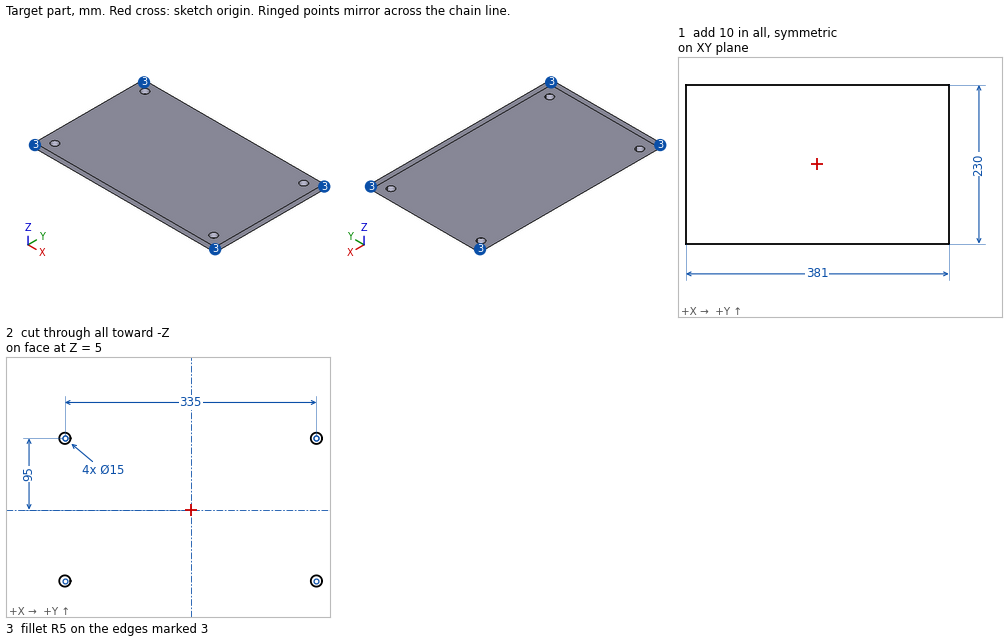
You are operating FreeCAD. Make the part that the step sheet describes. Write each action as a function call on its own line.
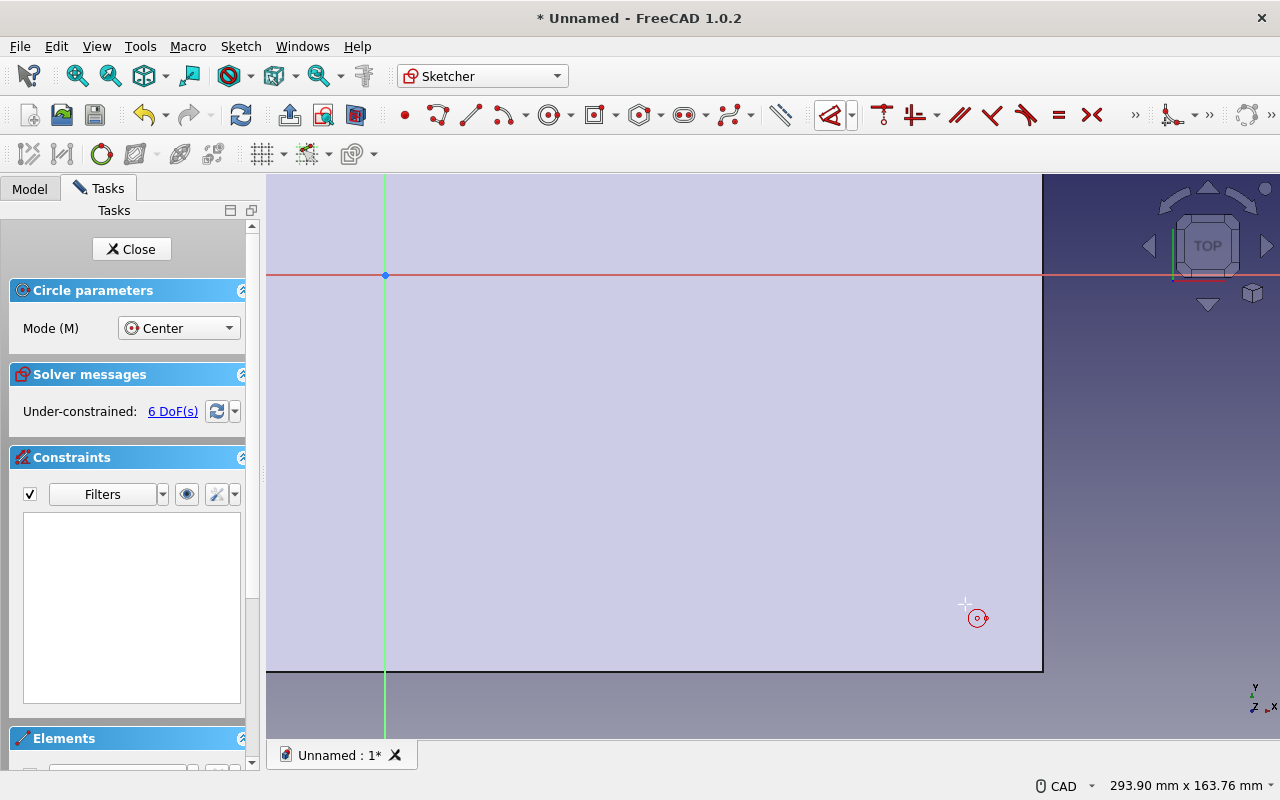
click(963, 603)
click(981, 585)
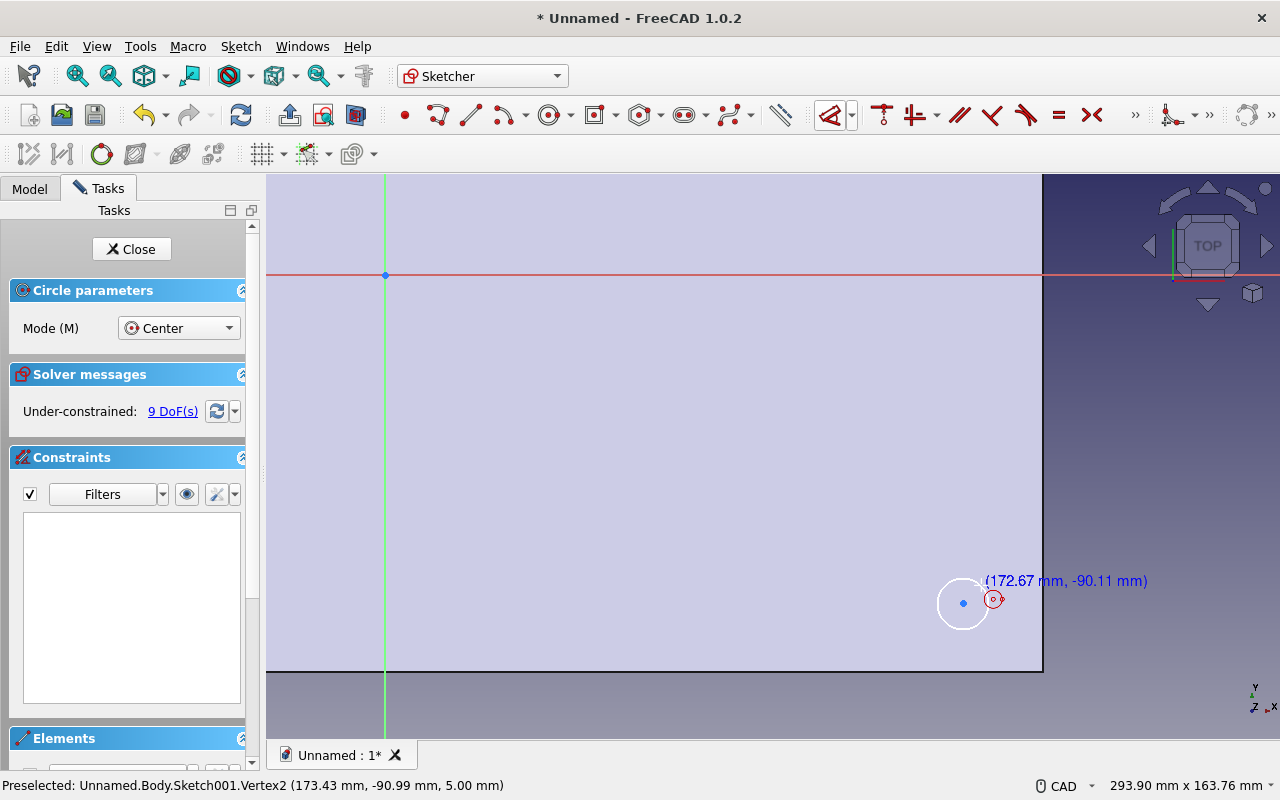
scroll(965, 605, down, 4)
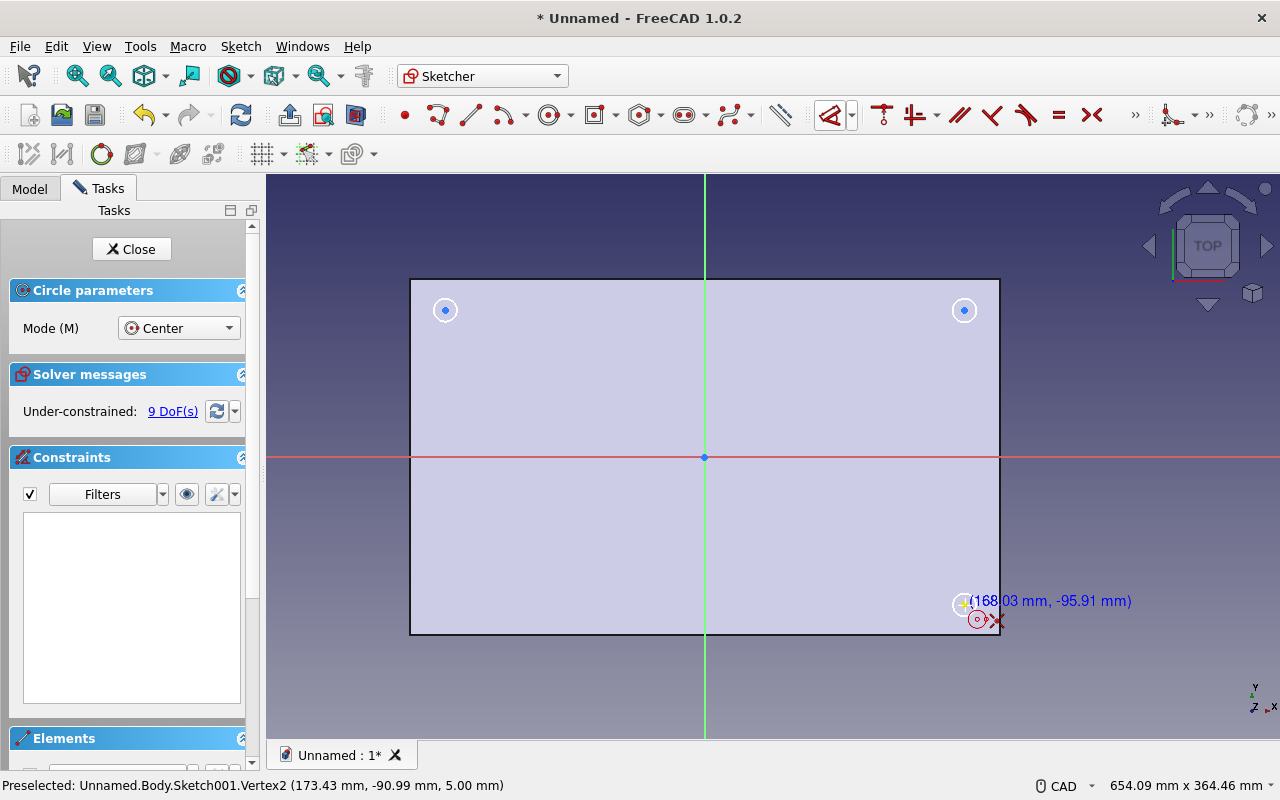
scroll(445, 604, up, 4)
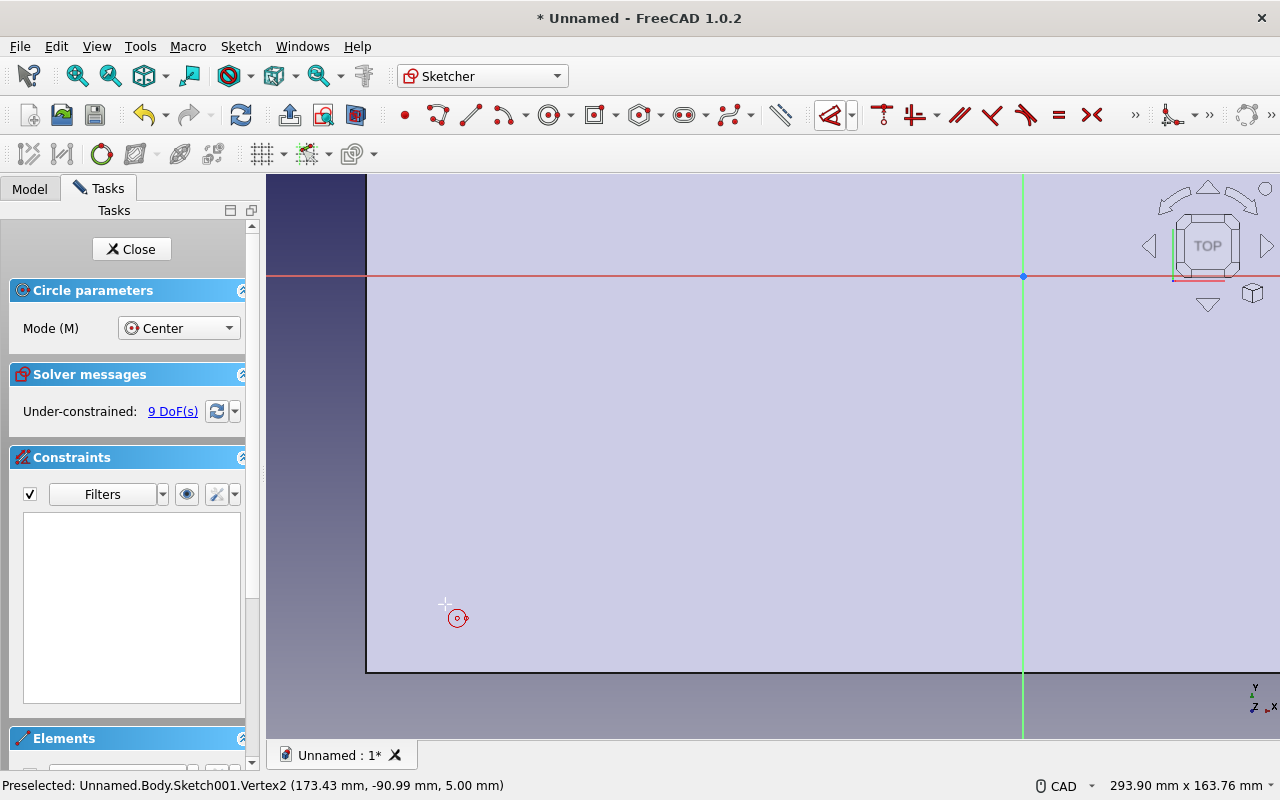
click(445, 604)
click(464, 586)
key(Escape)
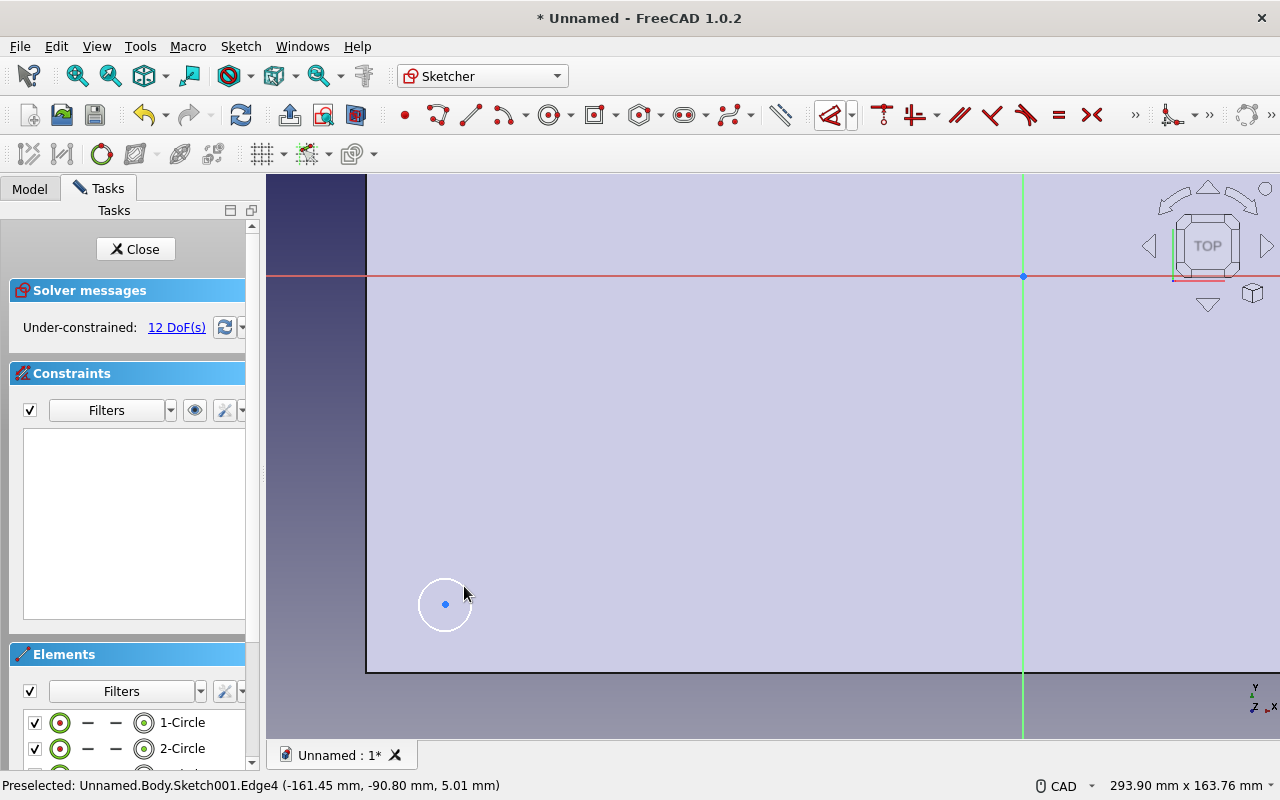
scroll(444, 604, down, 4)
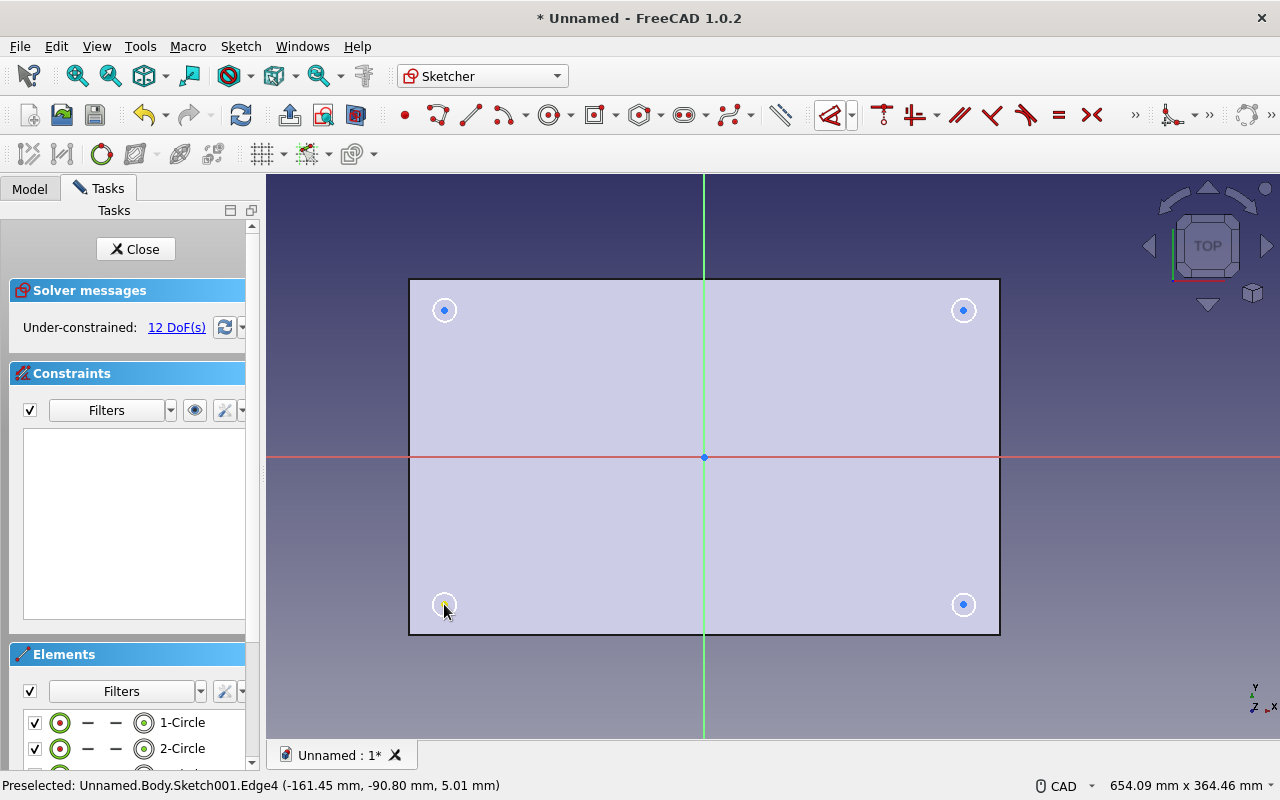
click(453, 302)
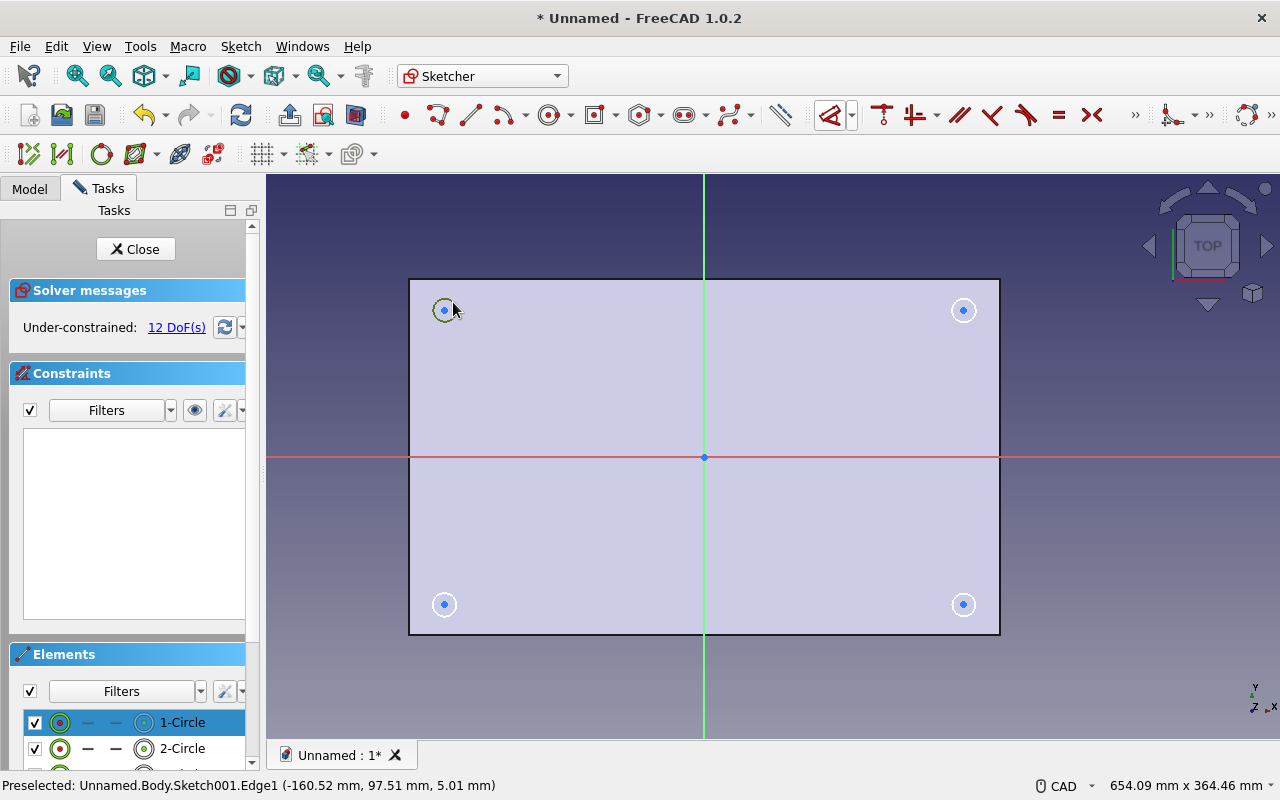
click(972, 302)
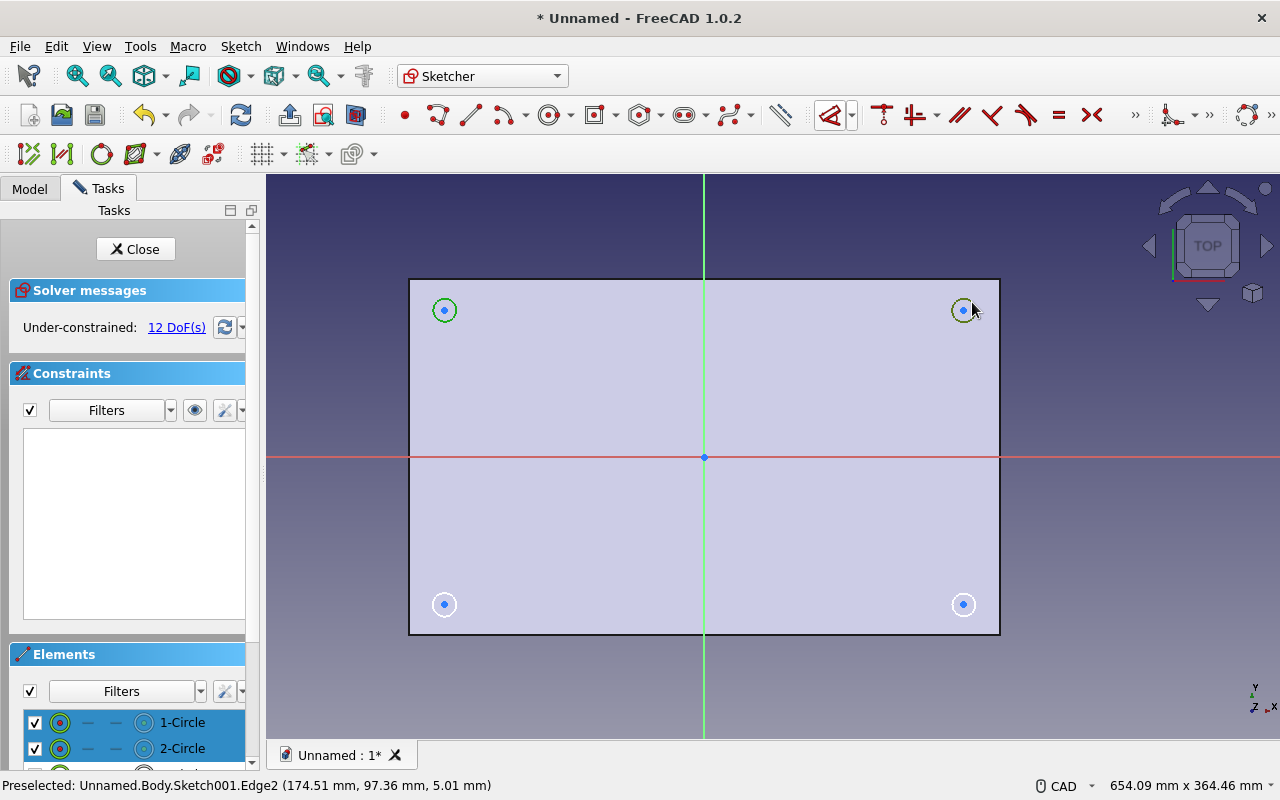
click(972, 597)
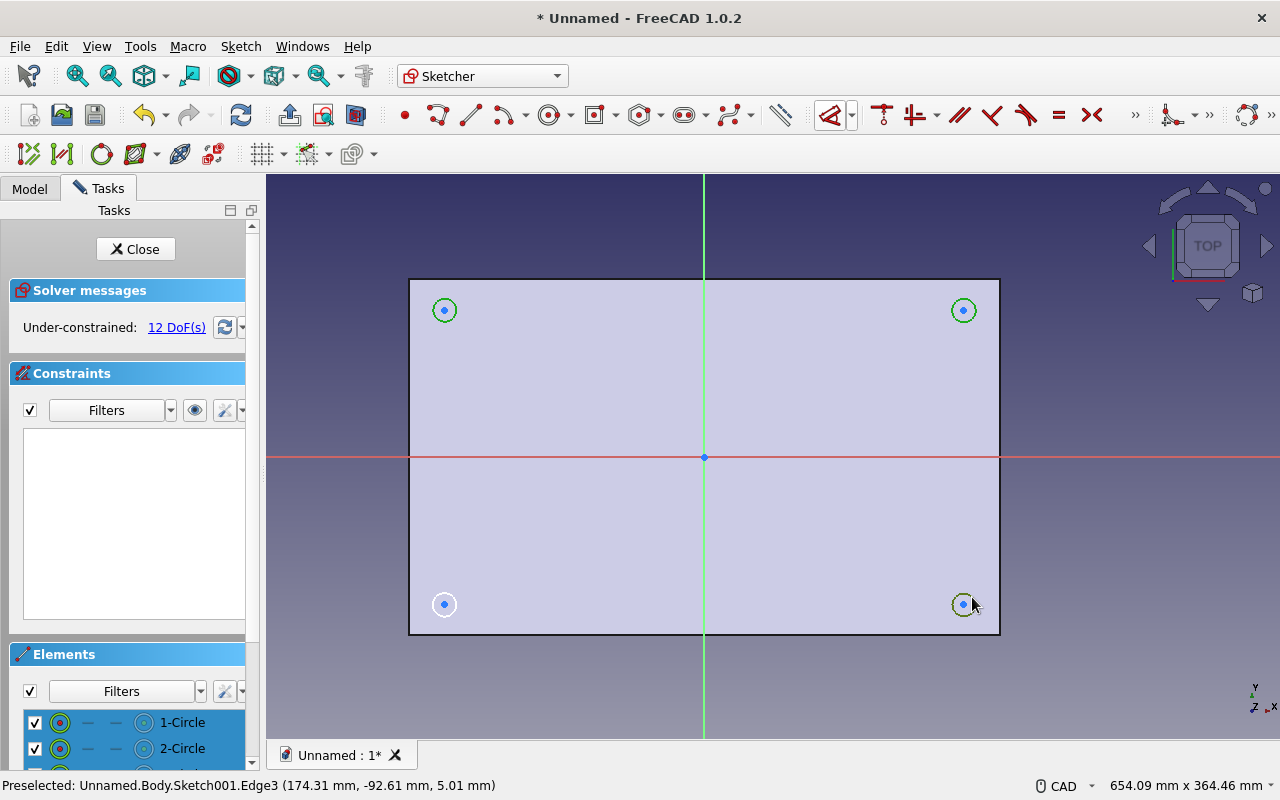
click(453, 597)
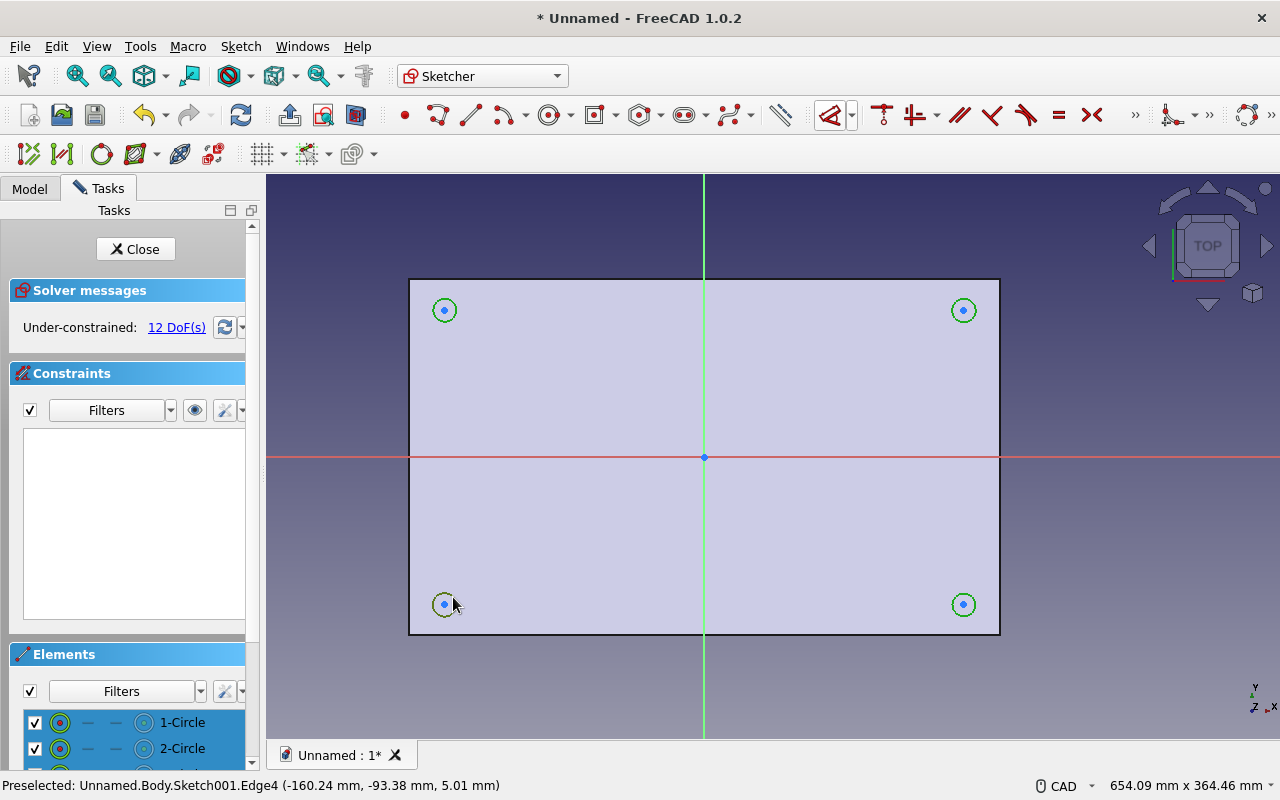
click(1059, 116)